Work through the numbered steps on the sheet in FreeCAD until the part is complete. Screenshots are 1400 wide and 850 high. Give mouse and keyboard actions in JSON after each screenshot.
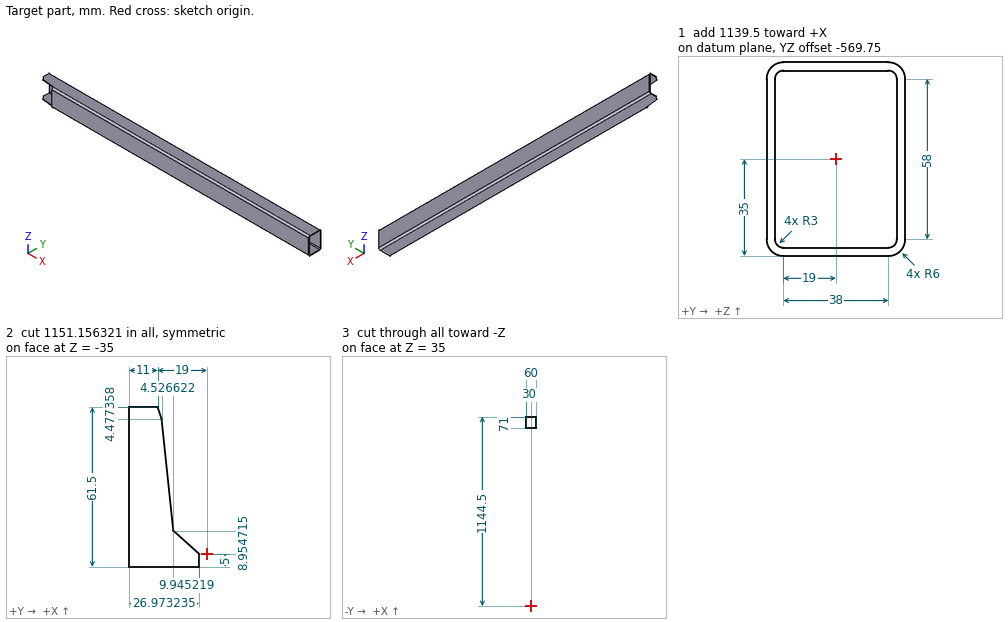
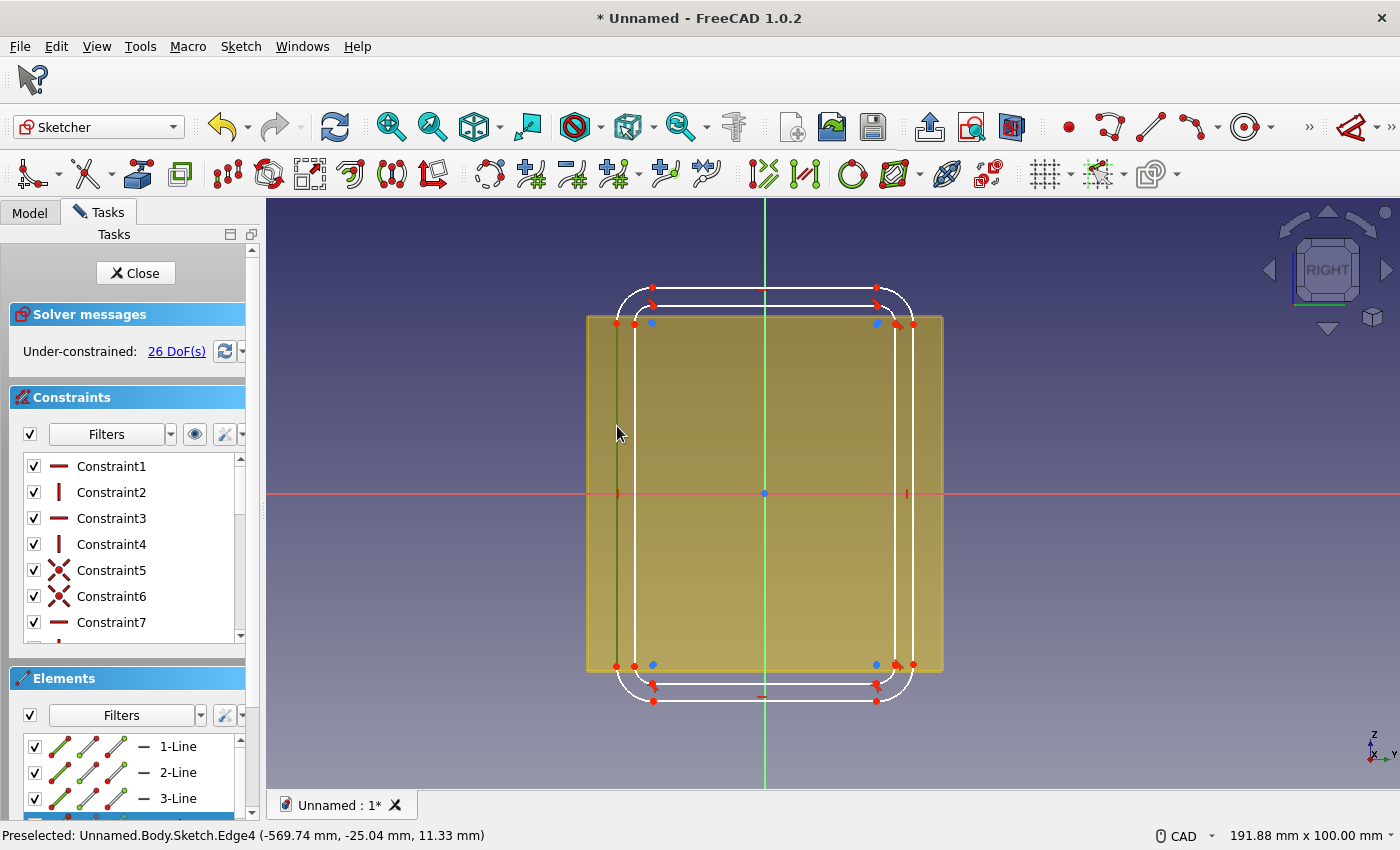
{"action": "left_click", "coordinate": [637, 292]}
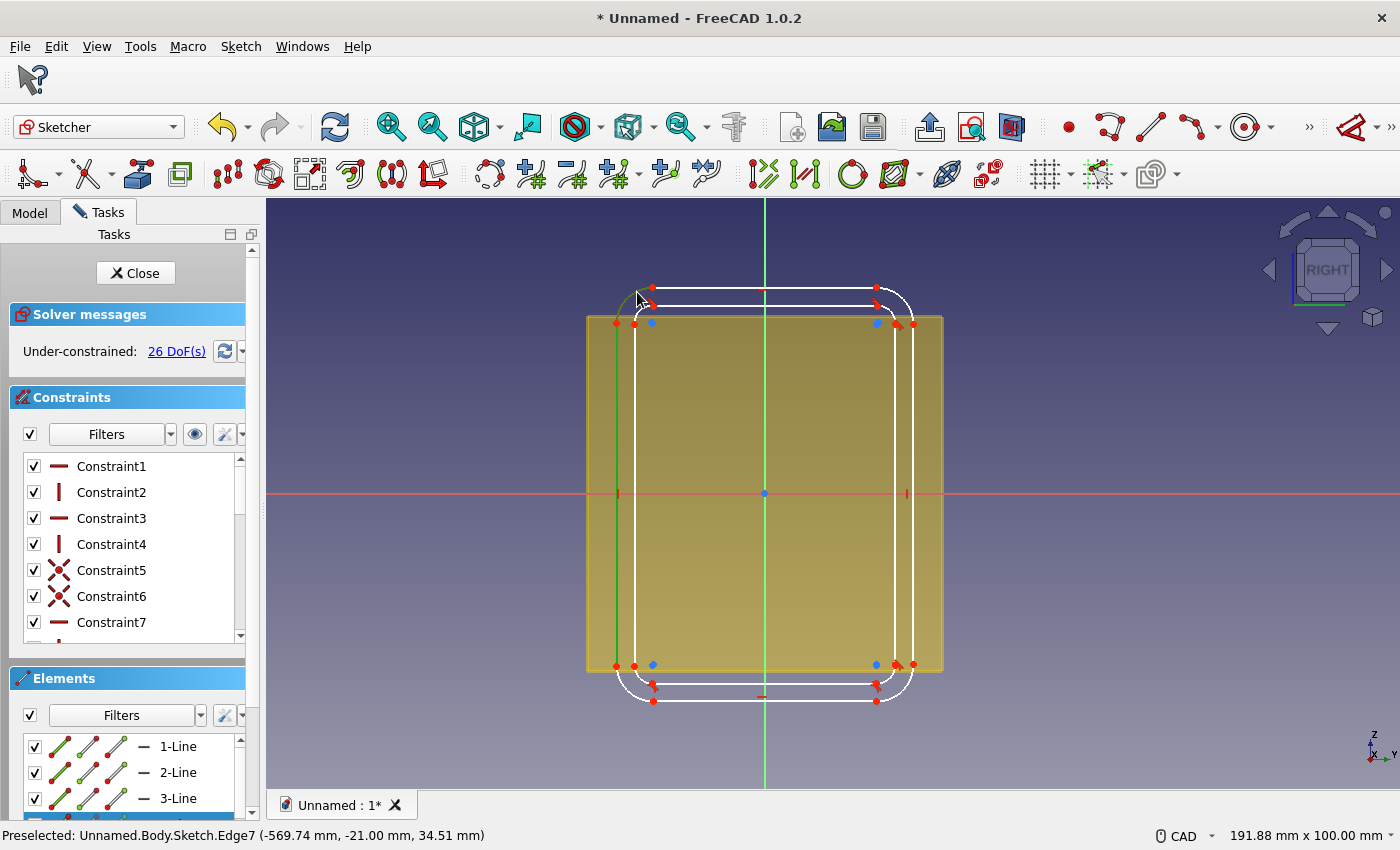
{"action": "key", "text": "t"}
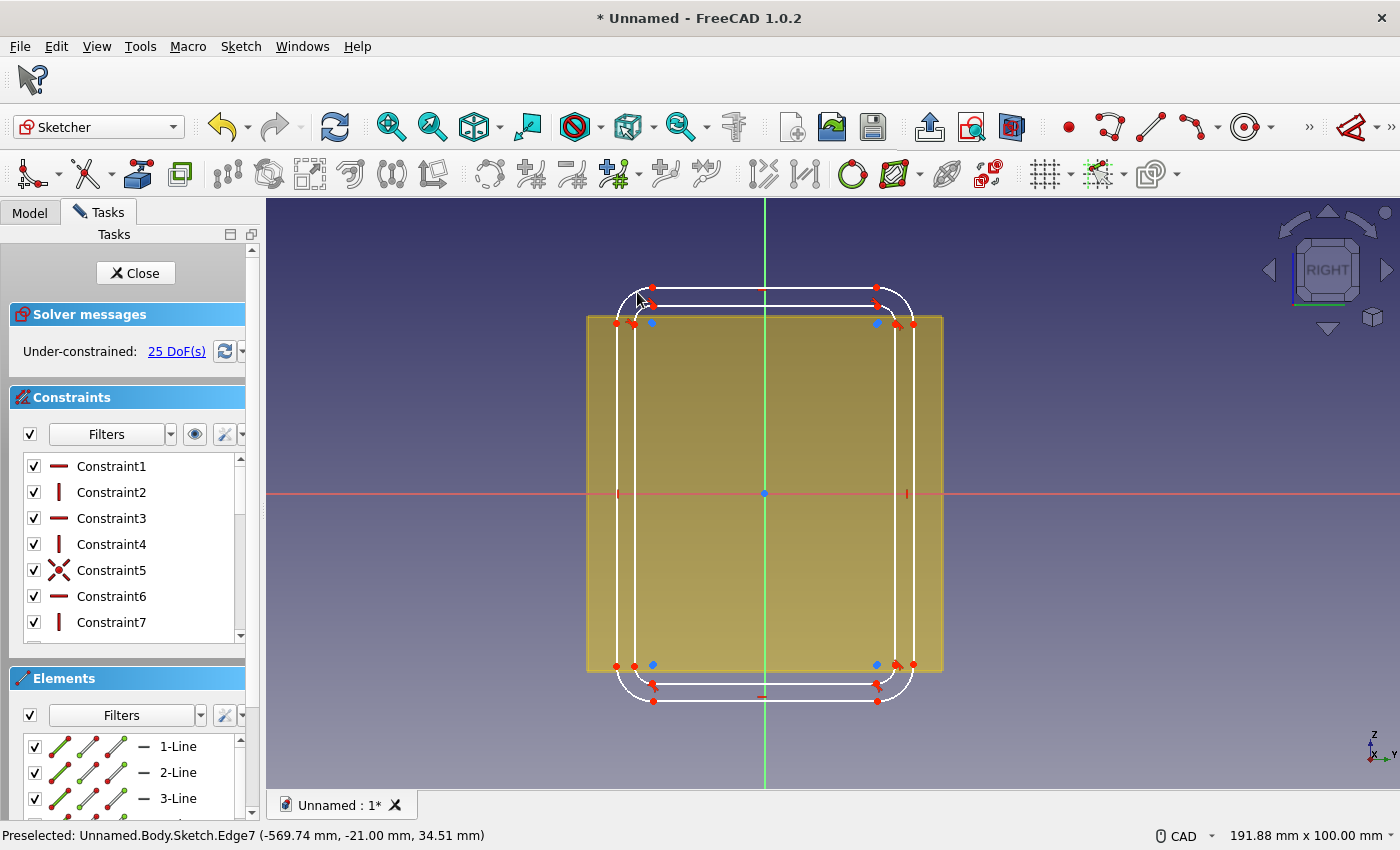
{"action": "left_click", "coordinate": [617, 426]}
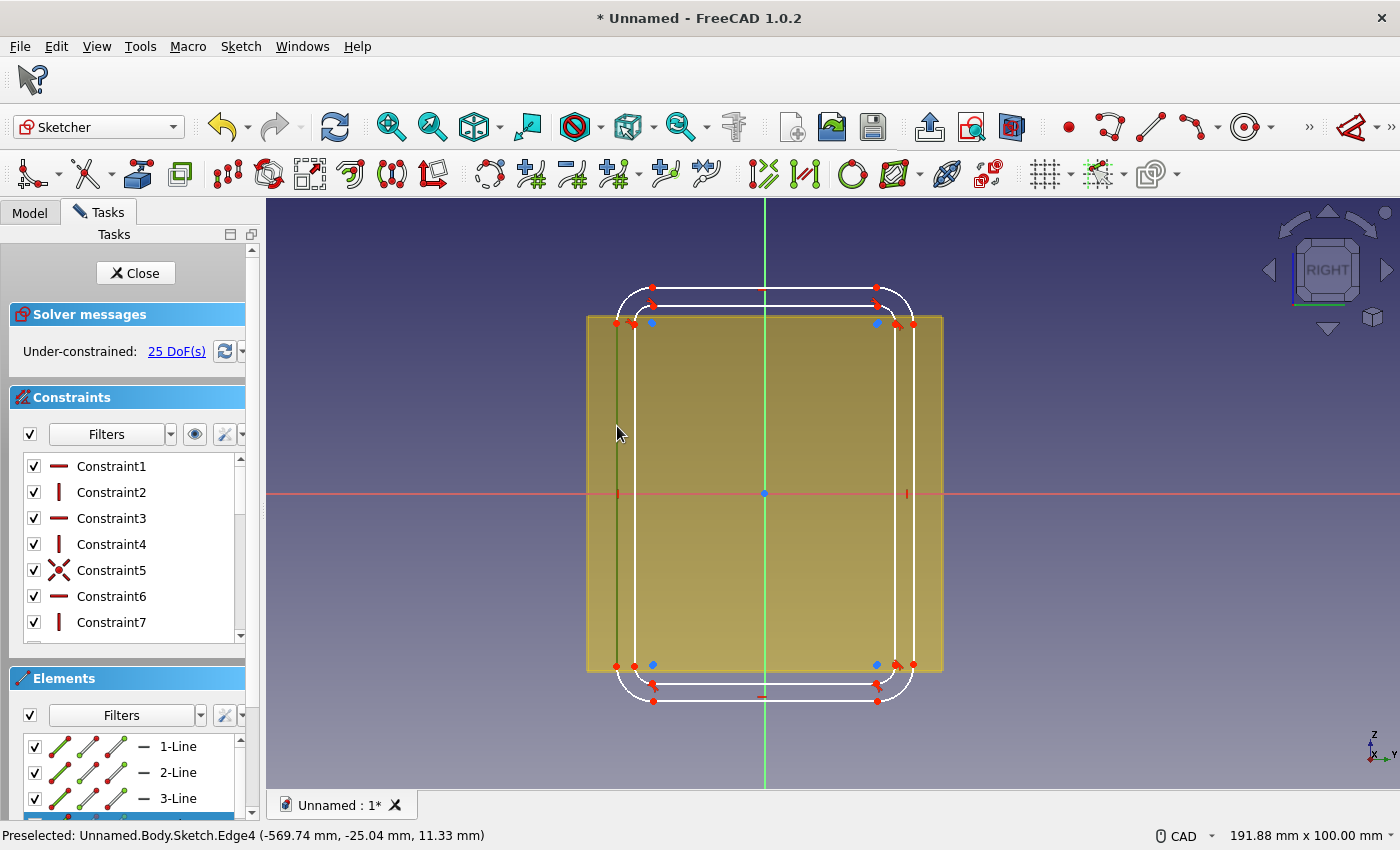
{"action": "left_click", "coordinate": [621, 682]}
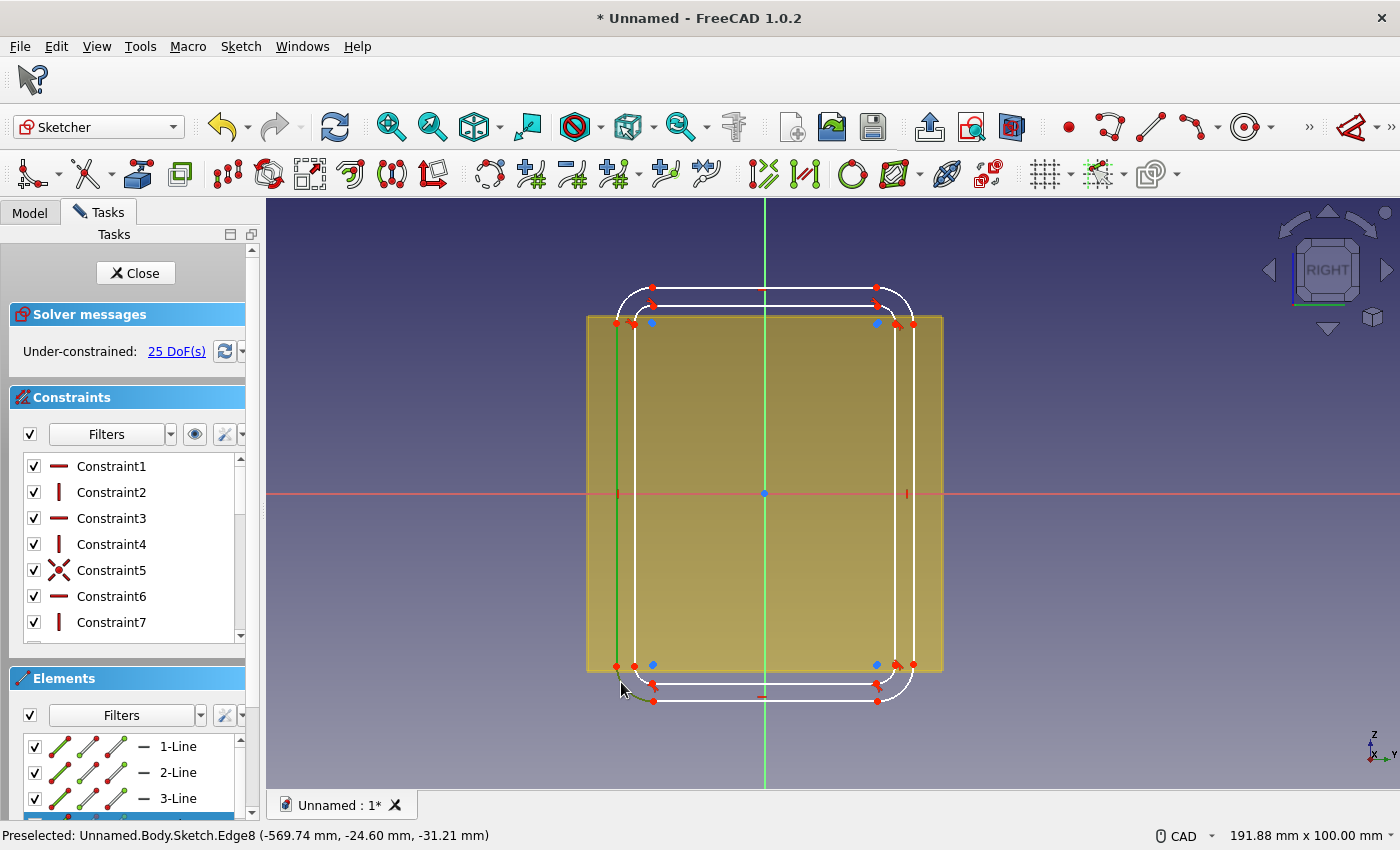
{"action": "key", "text": "t"}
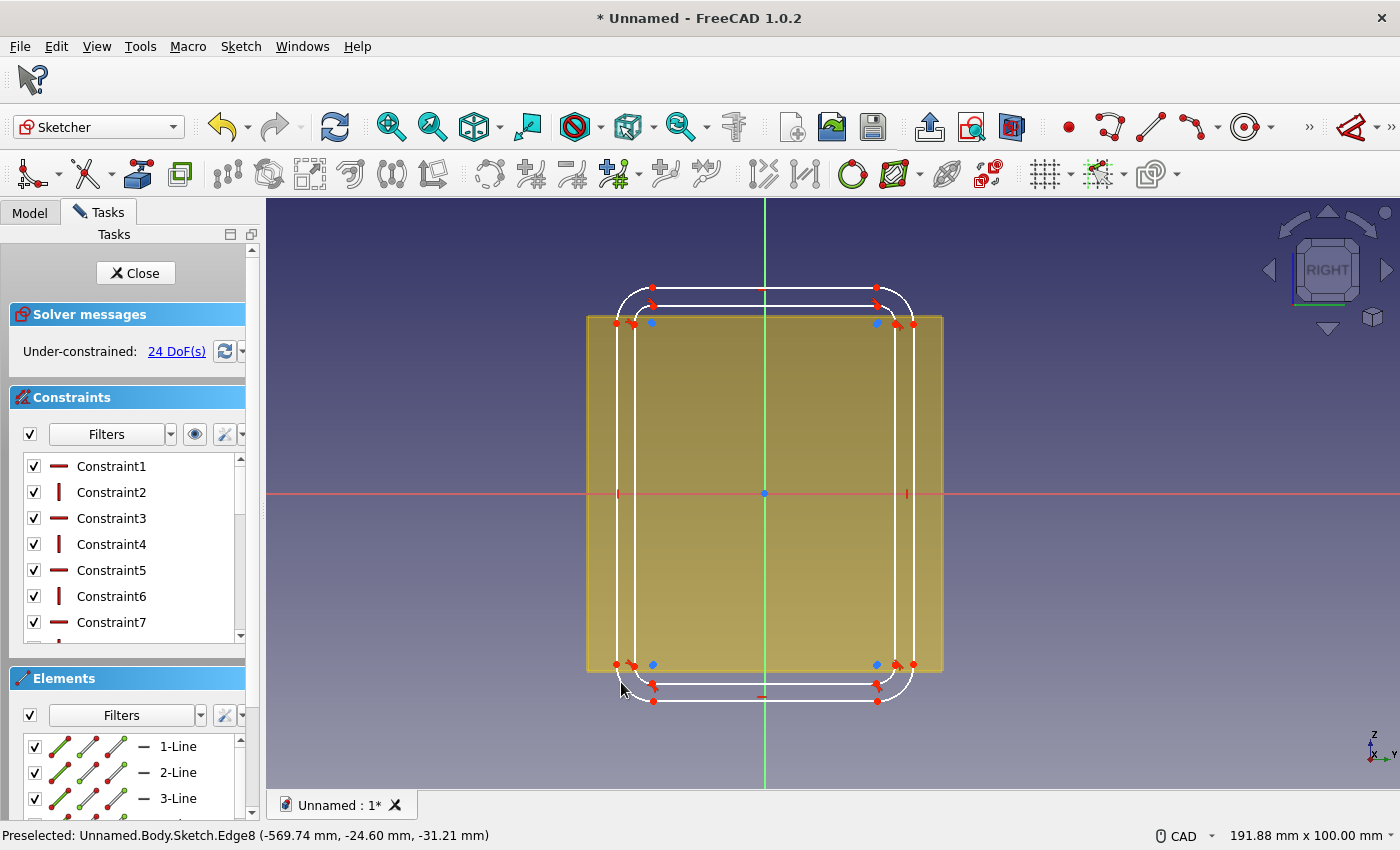
{"action": "left_click", "coordinate": [810, 684]}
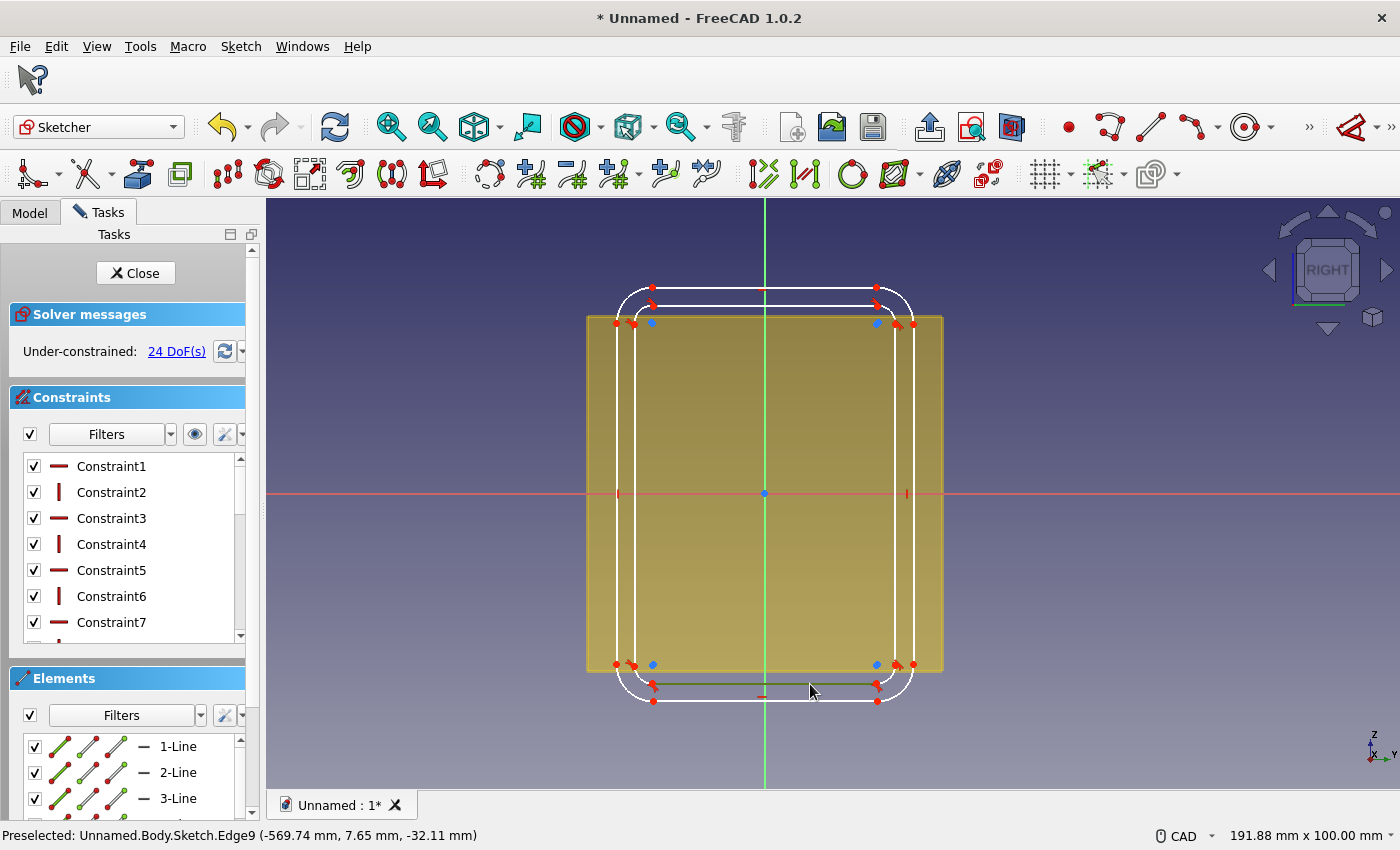
{"action": "left_click", "coordinate": [640, 678]}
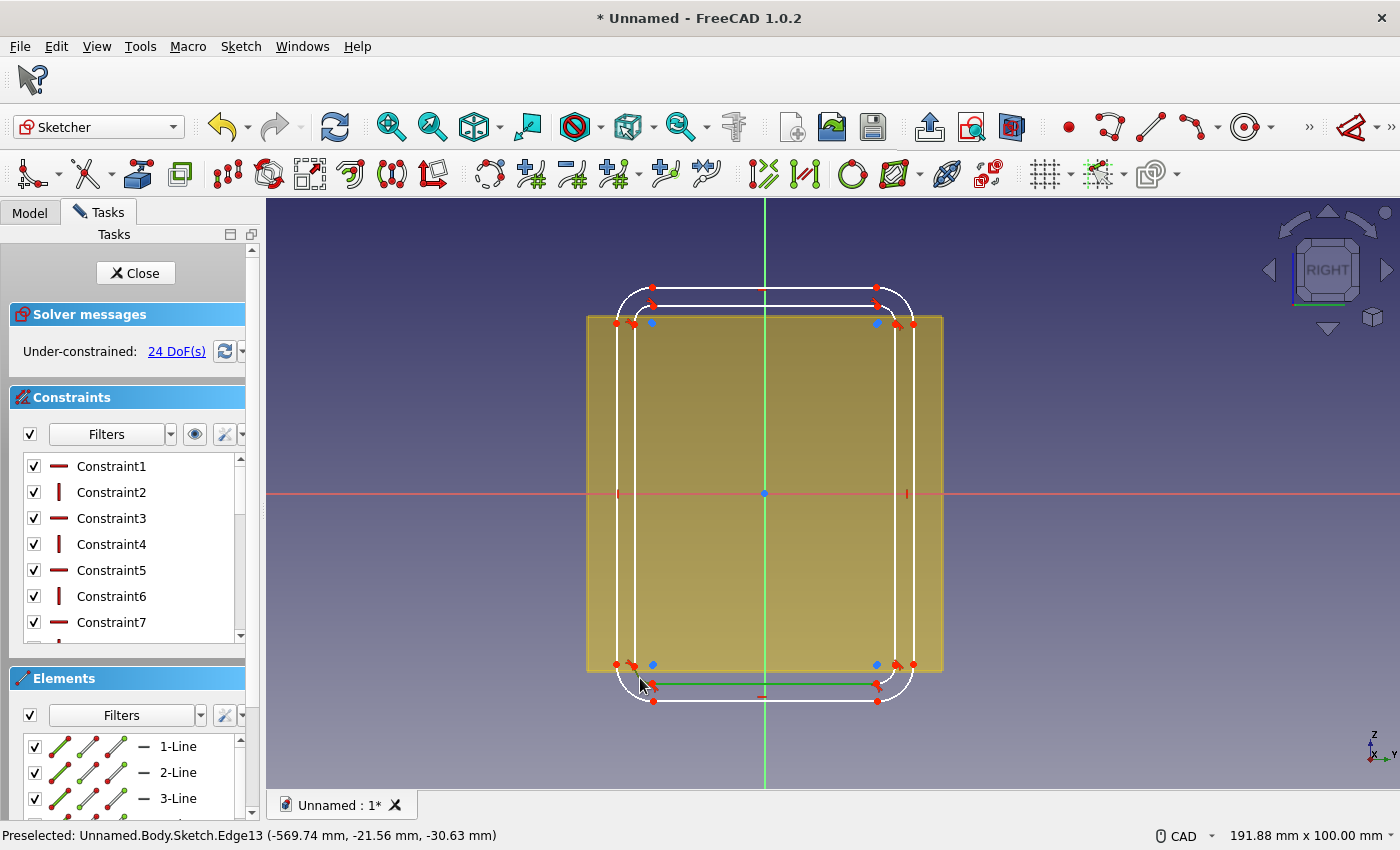
{"action": "key", "text": "t"}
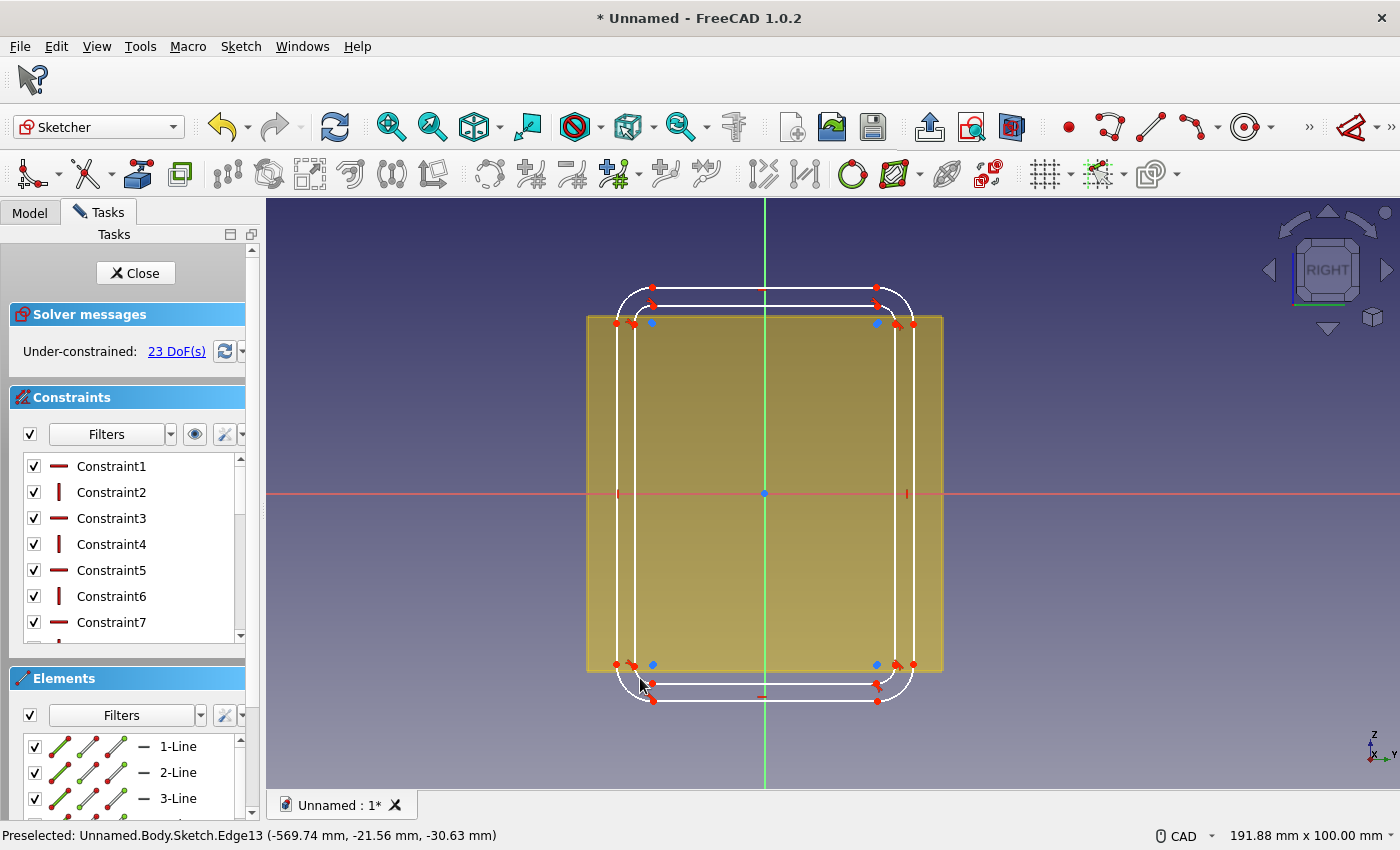
{"action": "left_click", "coordinate": [810, 684]}